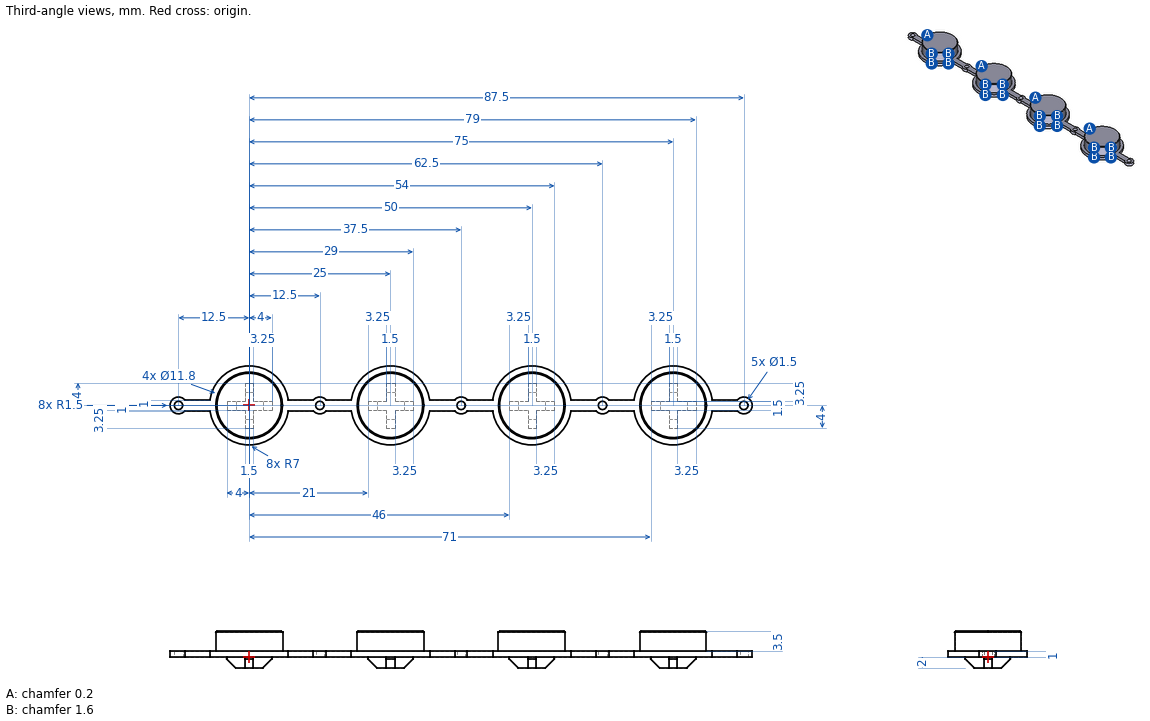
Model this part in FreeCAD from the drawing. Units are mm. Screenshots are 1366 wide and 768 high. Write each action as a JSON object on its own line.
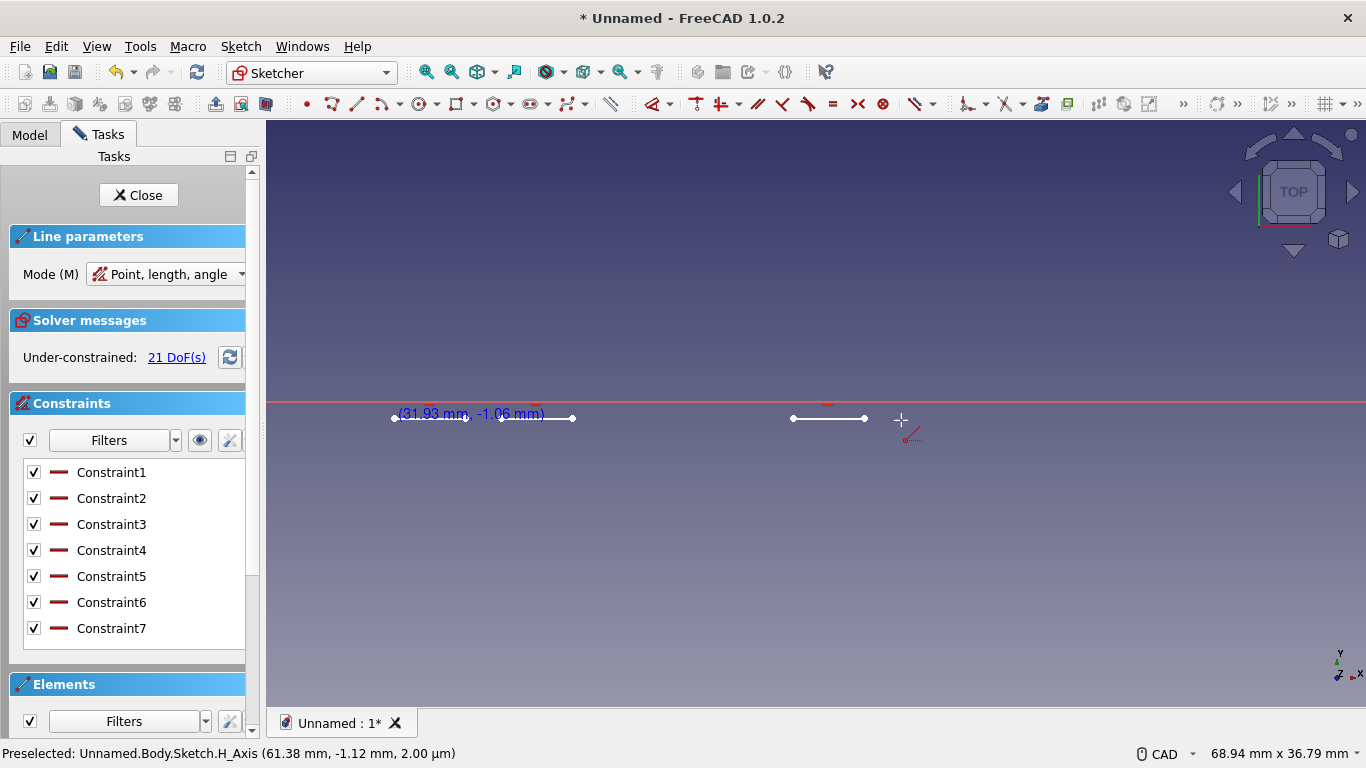
{"action": "left_click", "coordinate": [900, 418]}
{"action": "left_click", "coordinate": [971, 418]}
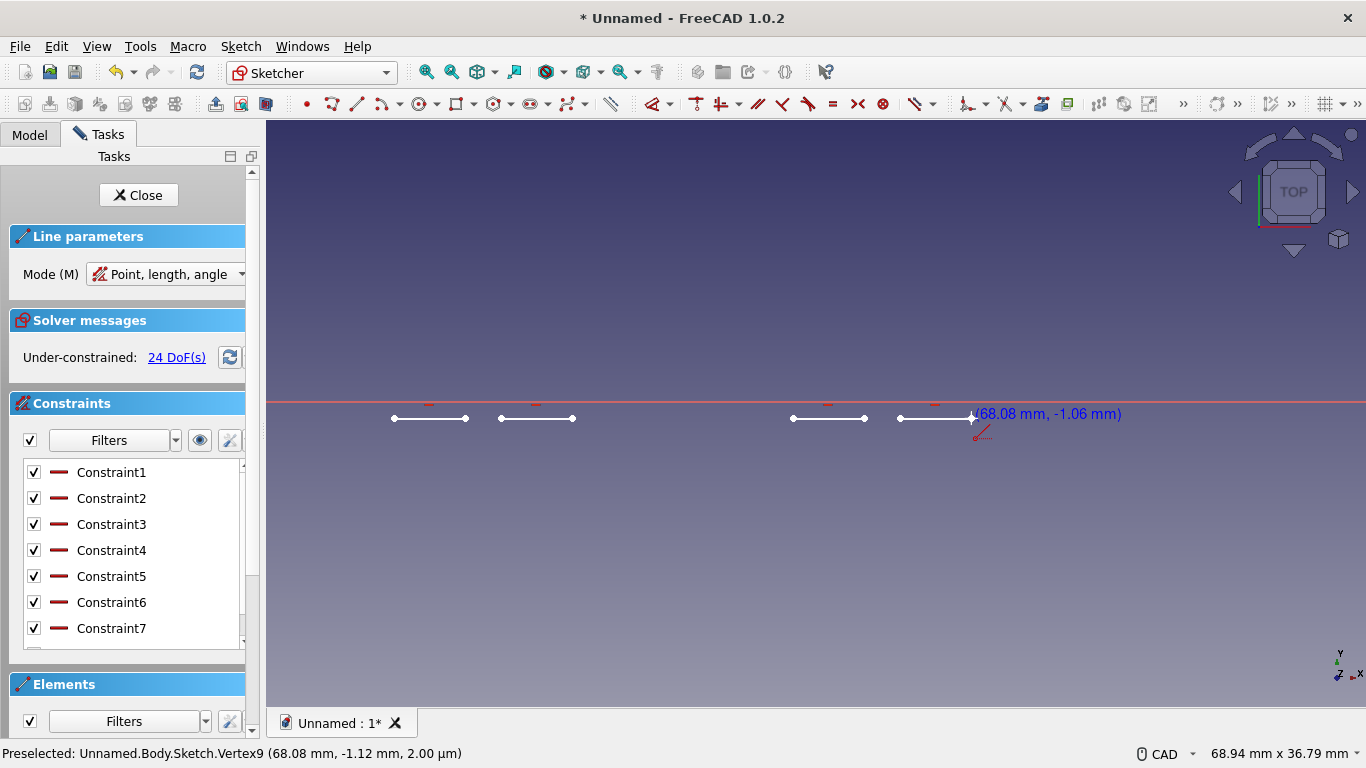
{"action": "left_click", "coordinate": [1192, 418]}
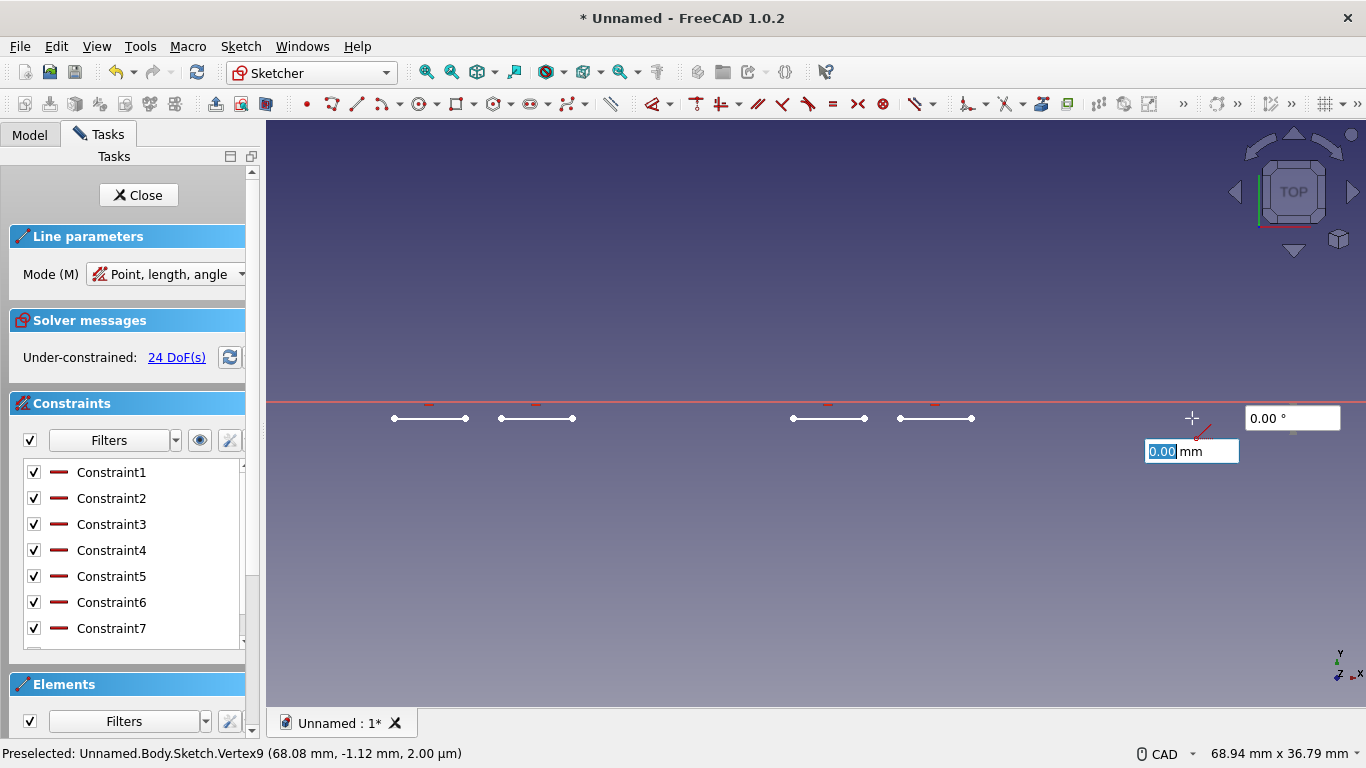
{"action": "scroll", "coordinate": [901, 420], "scroll_direction": "down", "scroll_amount": 5}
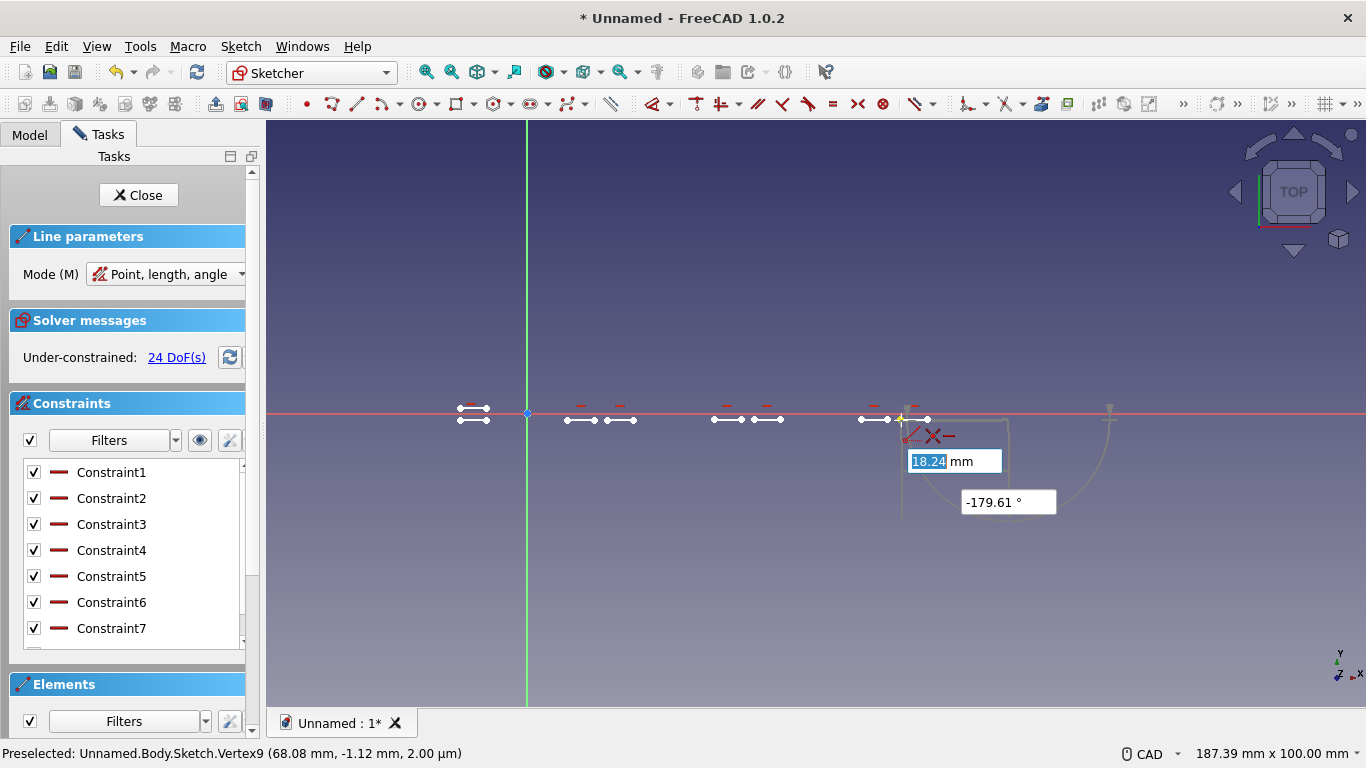
{"action": "scroll", "coordinate": [1035, 420], "scroll_direction": "up", "scroll_amount": 5}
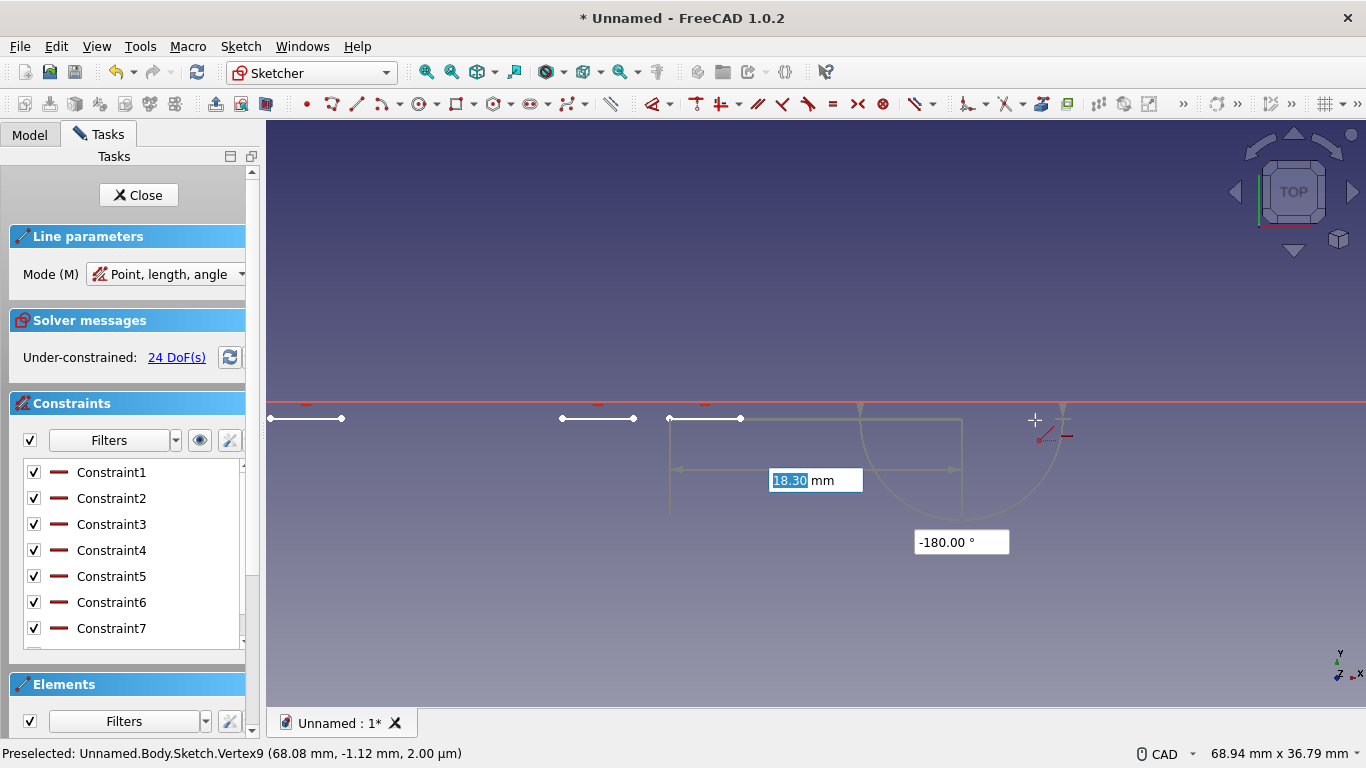
{"action": "left_click", "coordinate": [1033, 418]}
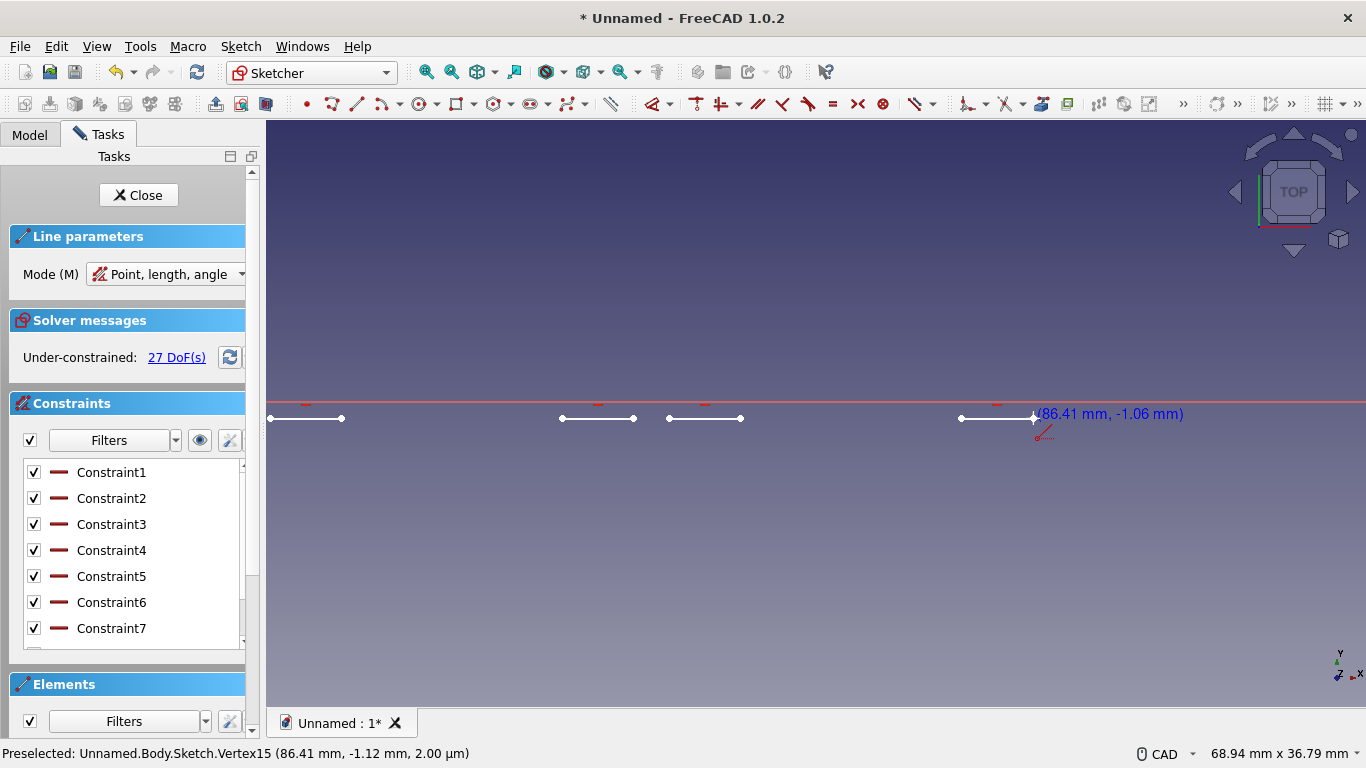
{"action": "left_click", "coordinate": [1033, 386]}
{"action": "left_click", "coordinate": [962, 386]}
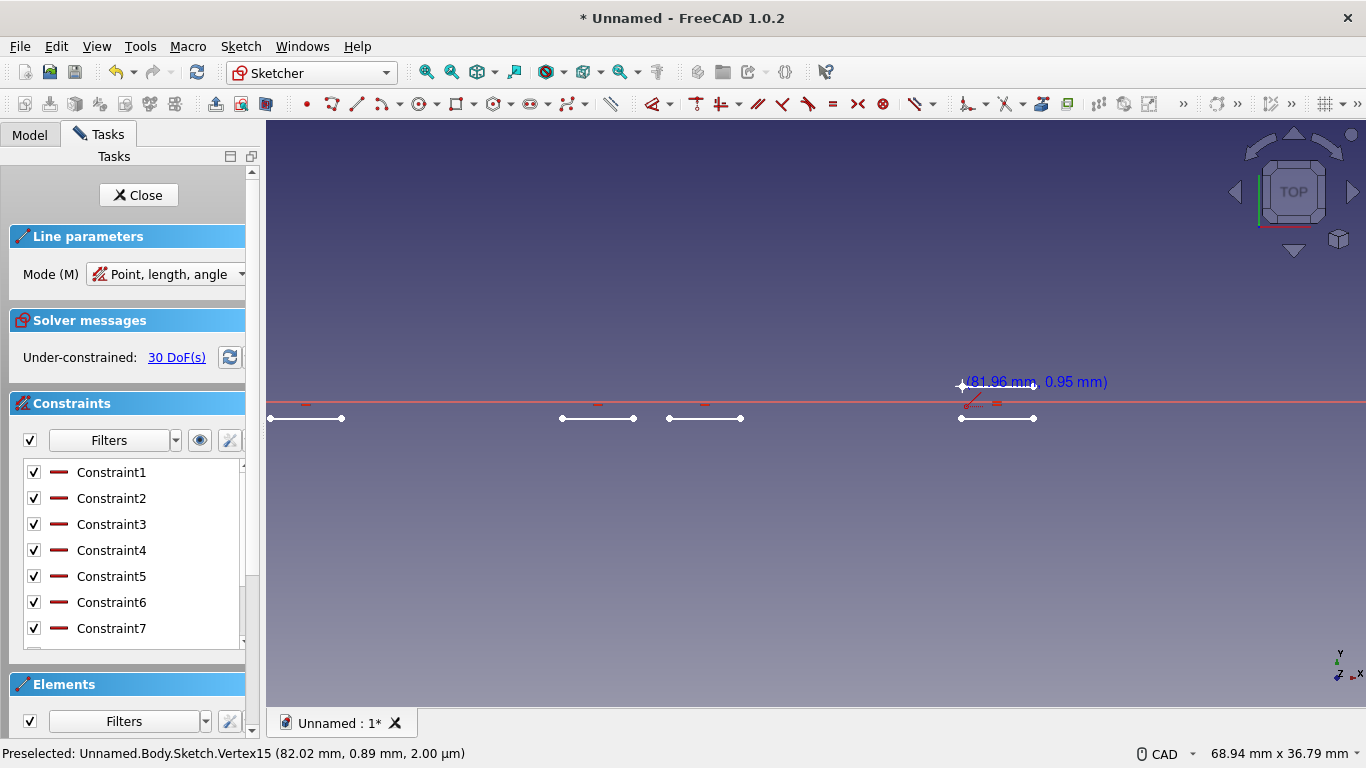
{"action": "left_click", "coordinate": [740, 386]}
{"action": "left_click", "coordinate": [669, 386]}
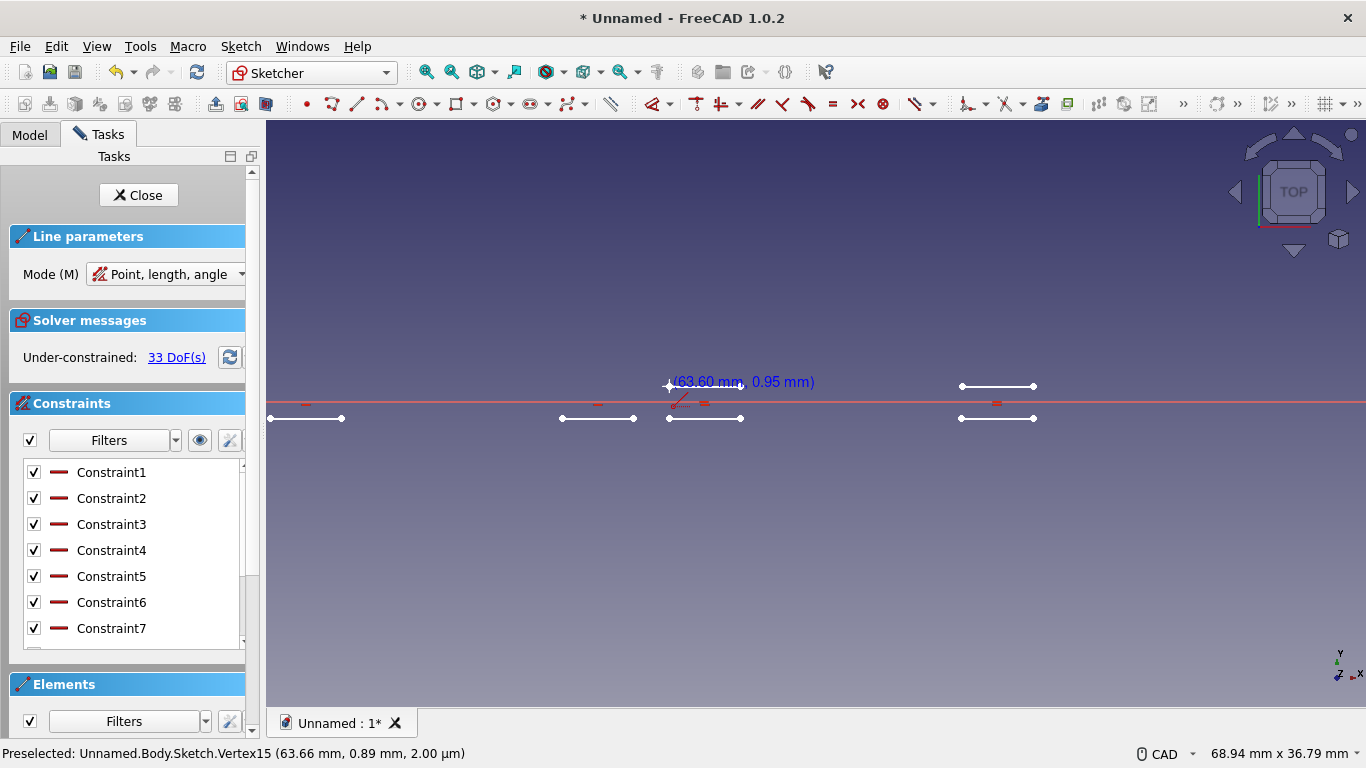
{"action": "left_click", "coordinate": [634, 386]}
{"action": "left_click", "coordinate": [563, 386]}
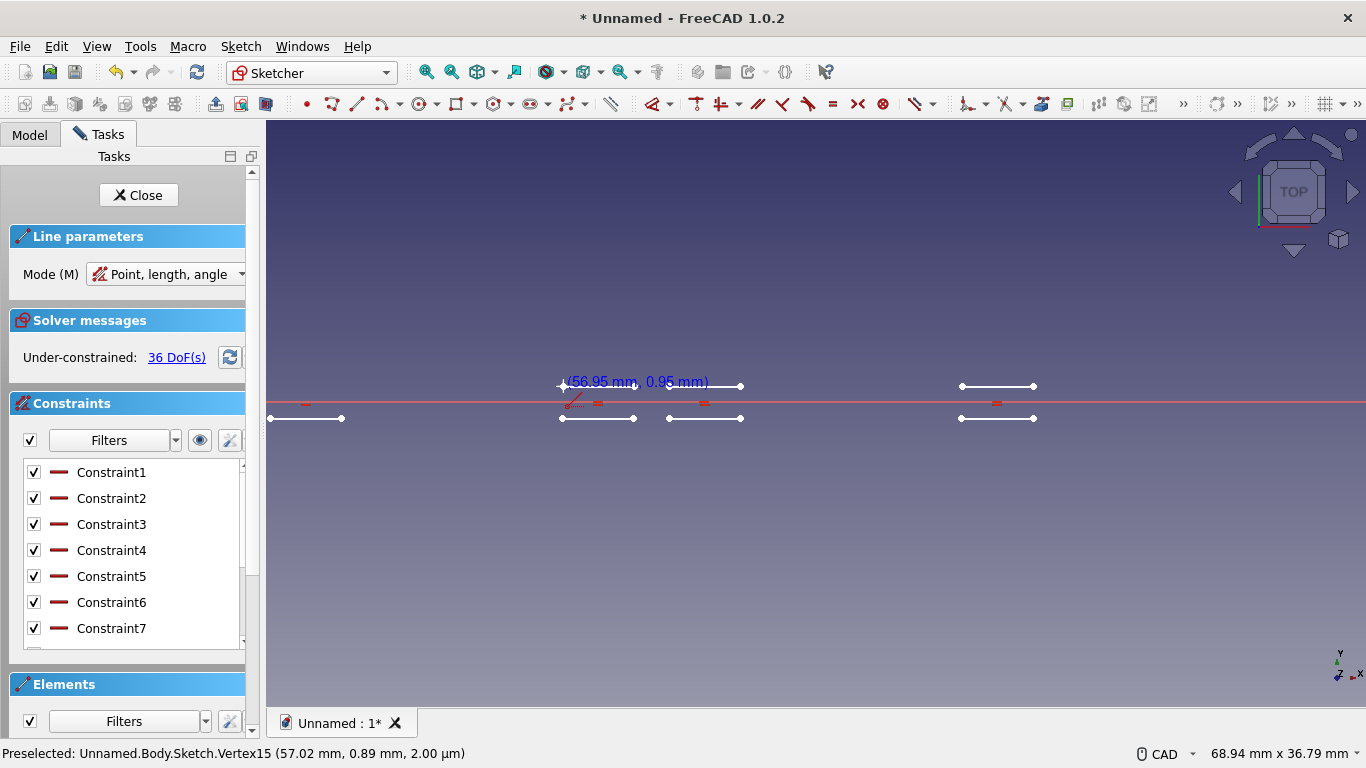
{"action": "left_click", "coordinate": [342, 386]}